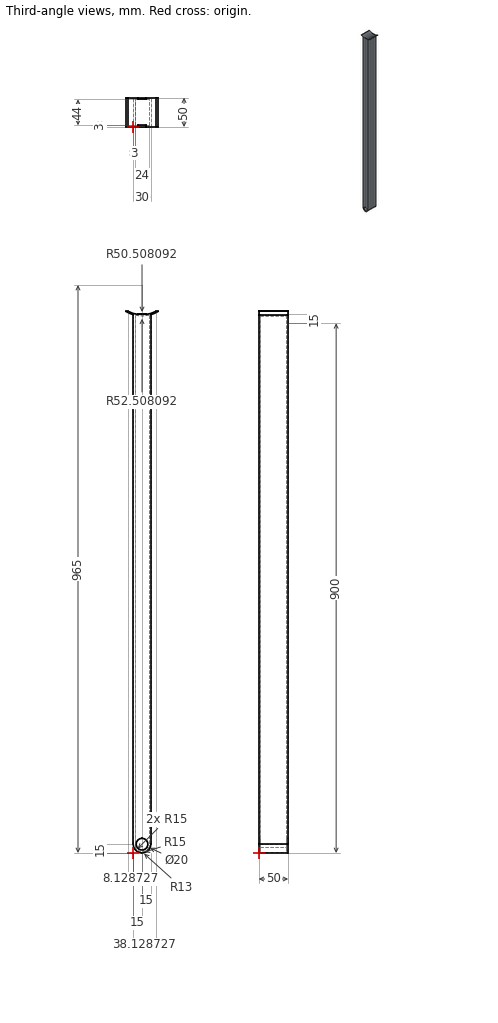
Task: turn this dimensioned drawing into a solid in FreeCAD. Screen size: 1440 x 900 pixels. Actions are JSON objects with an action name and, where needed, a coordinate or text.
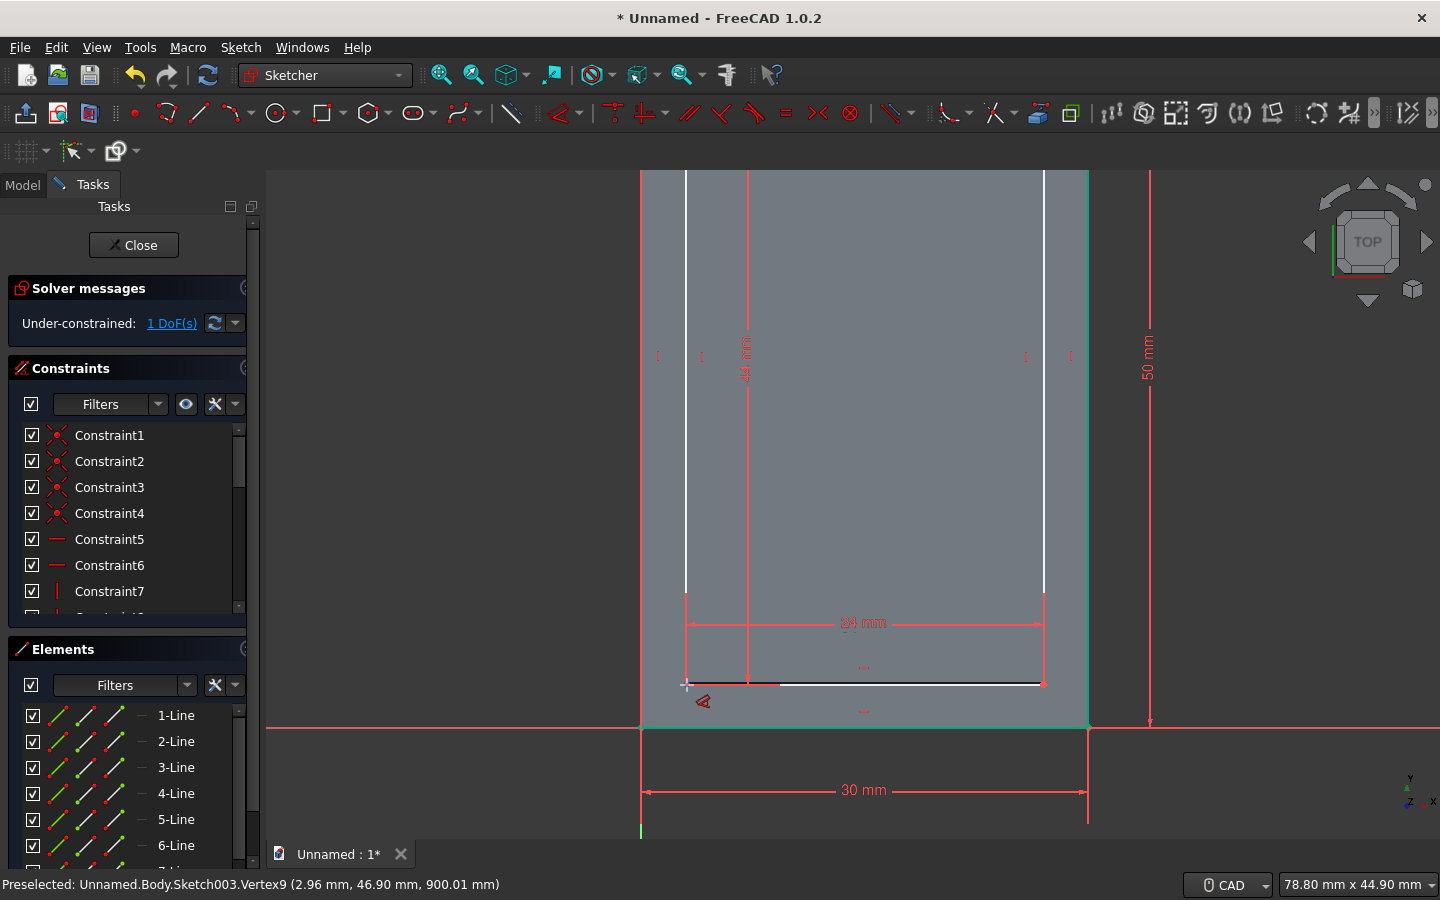
{"action": "left_click", "coordinate": [686, 685]}
{"action": "left_click", "coordinate": [607, 706]}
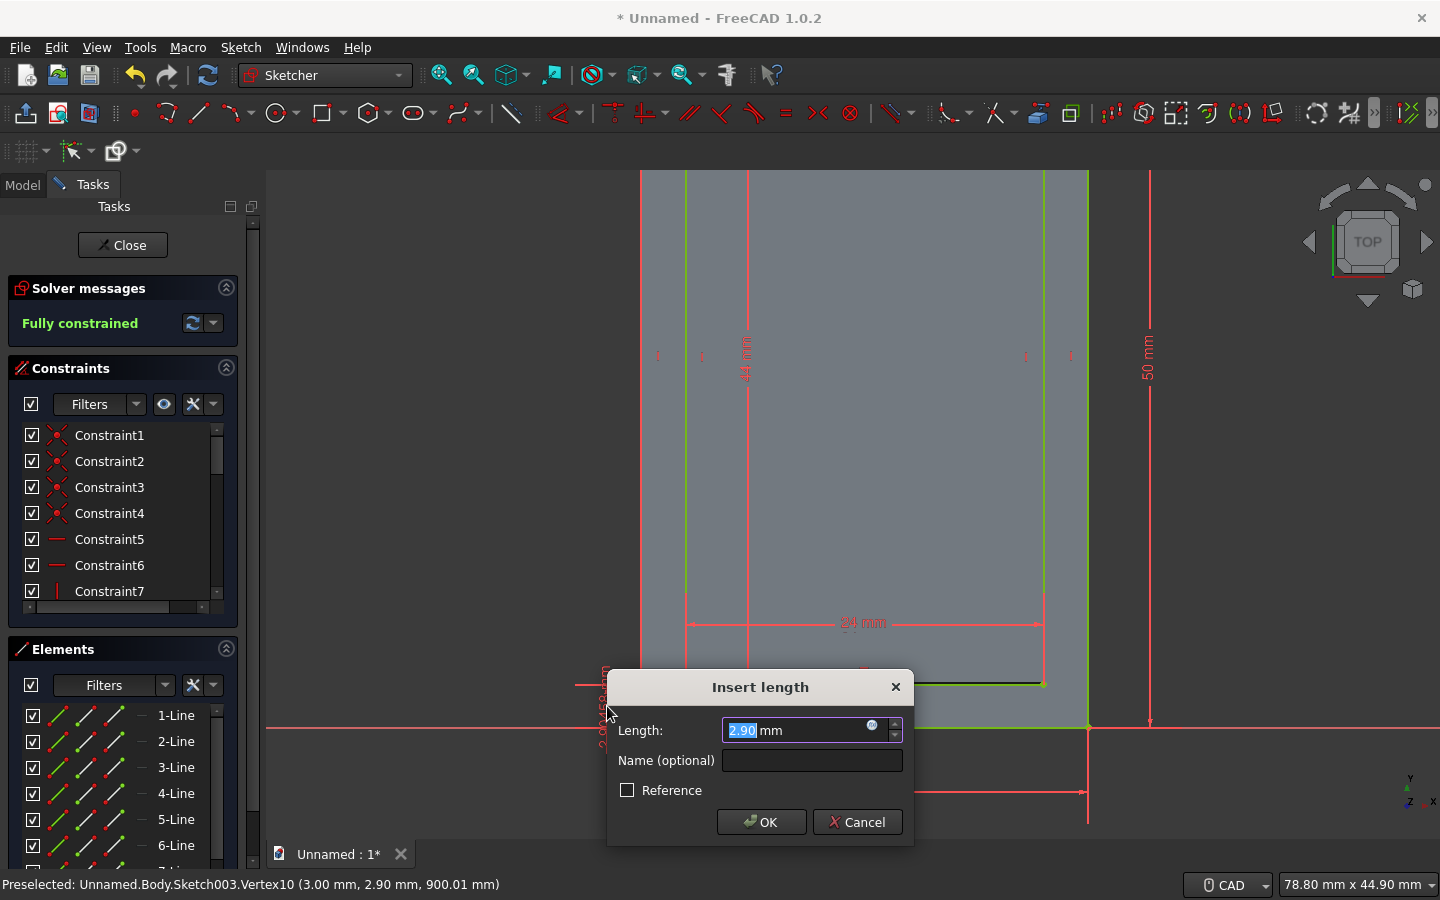
{"action": "type", "text": "3"}
{"action": "key", "text": "Return"}
{"action": "key", "text": "Escape"}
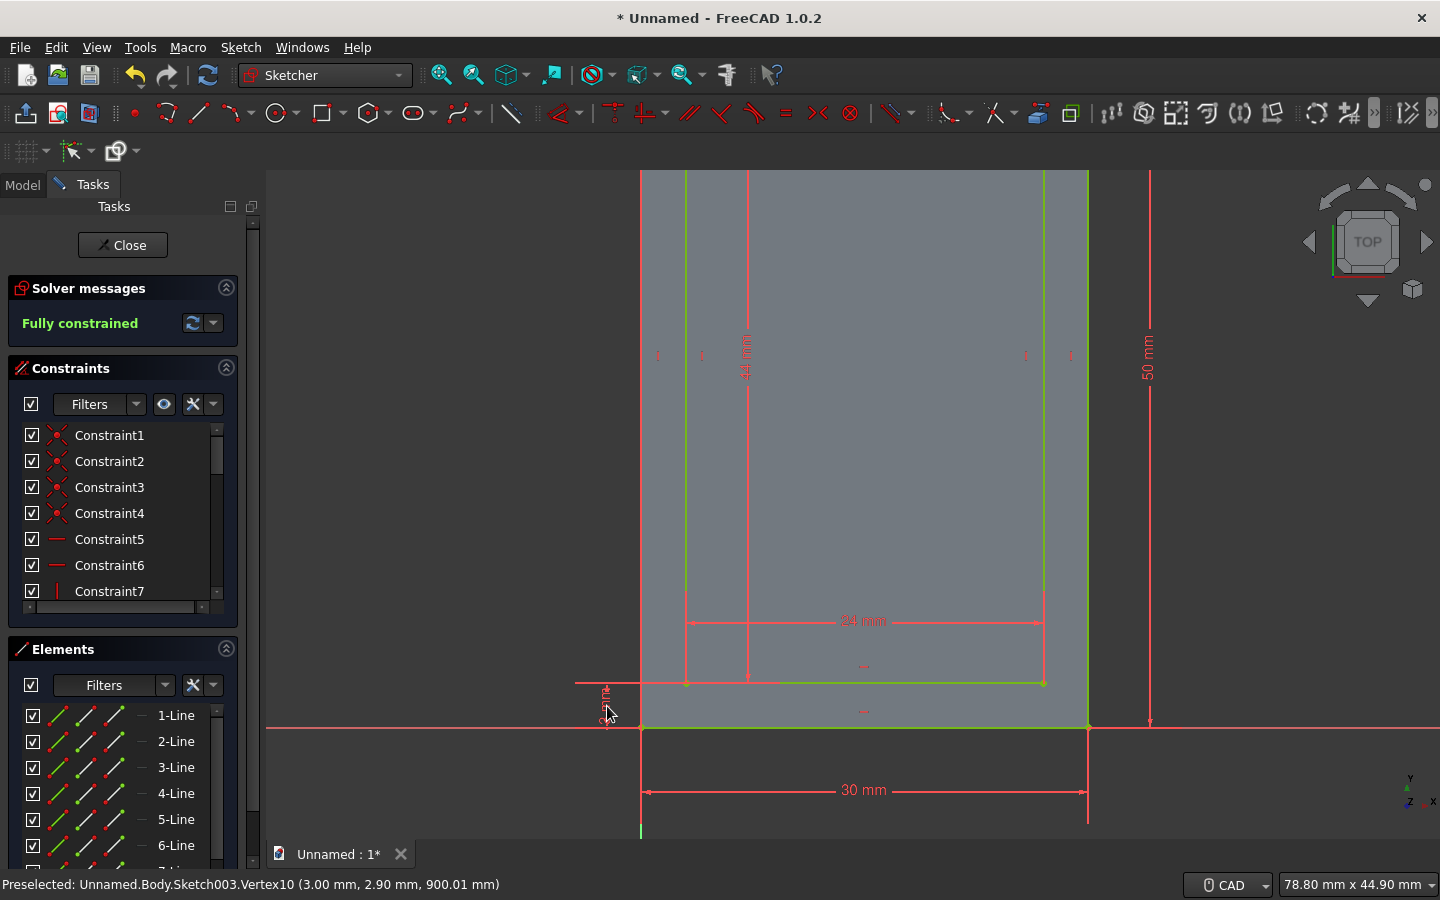
{"action": "left_click", "coordinate": [123, 245]}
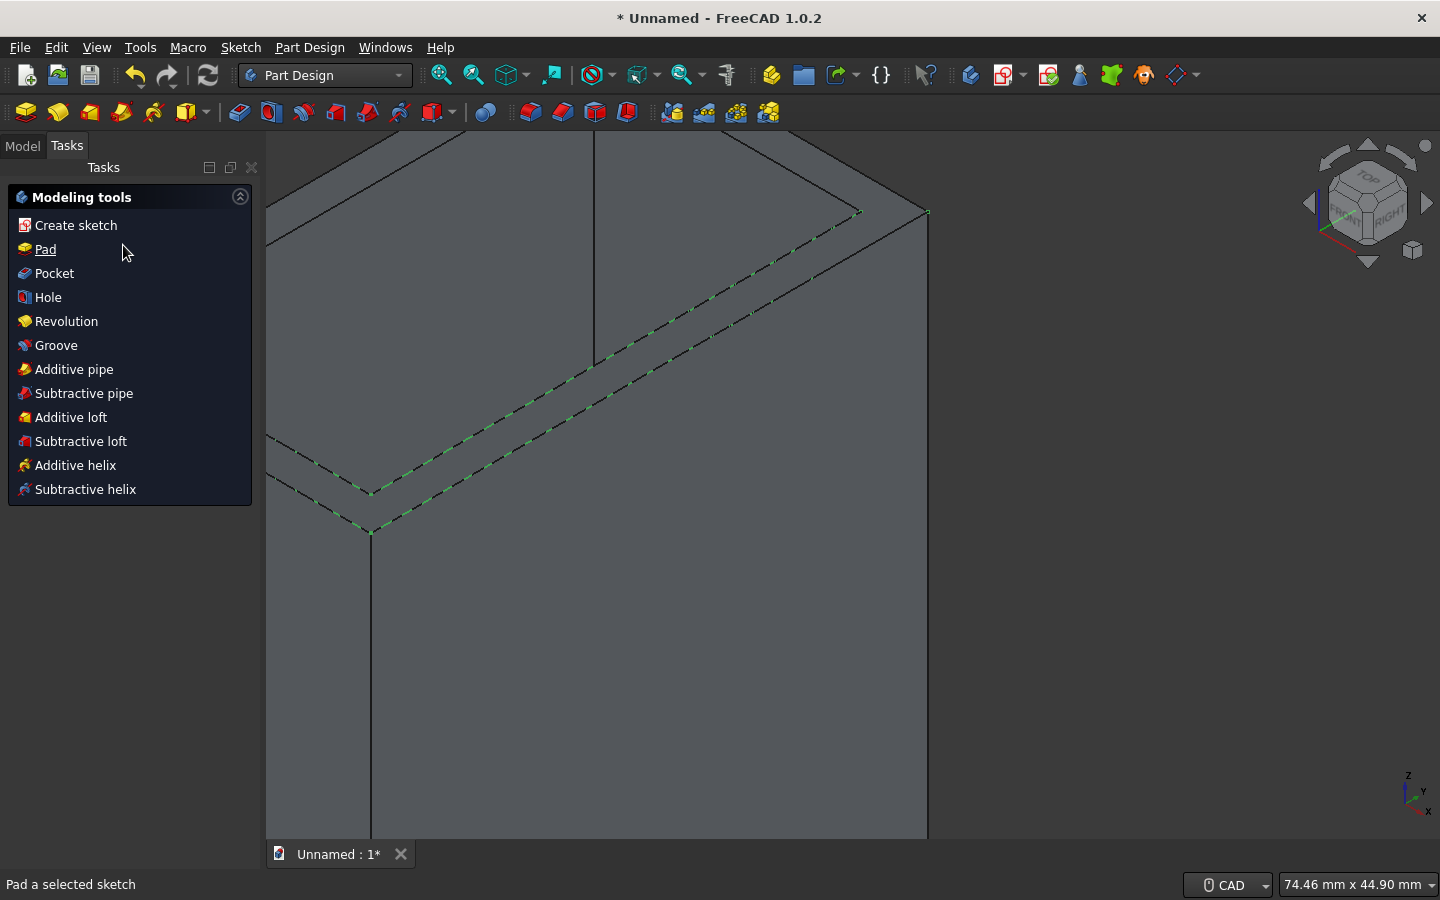
{"action": "left_click", "coordinate": [26, 112]}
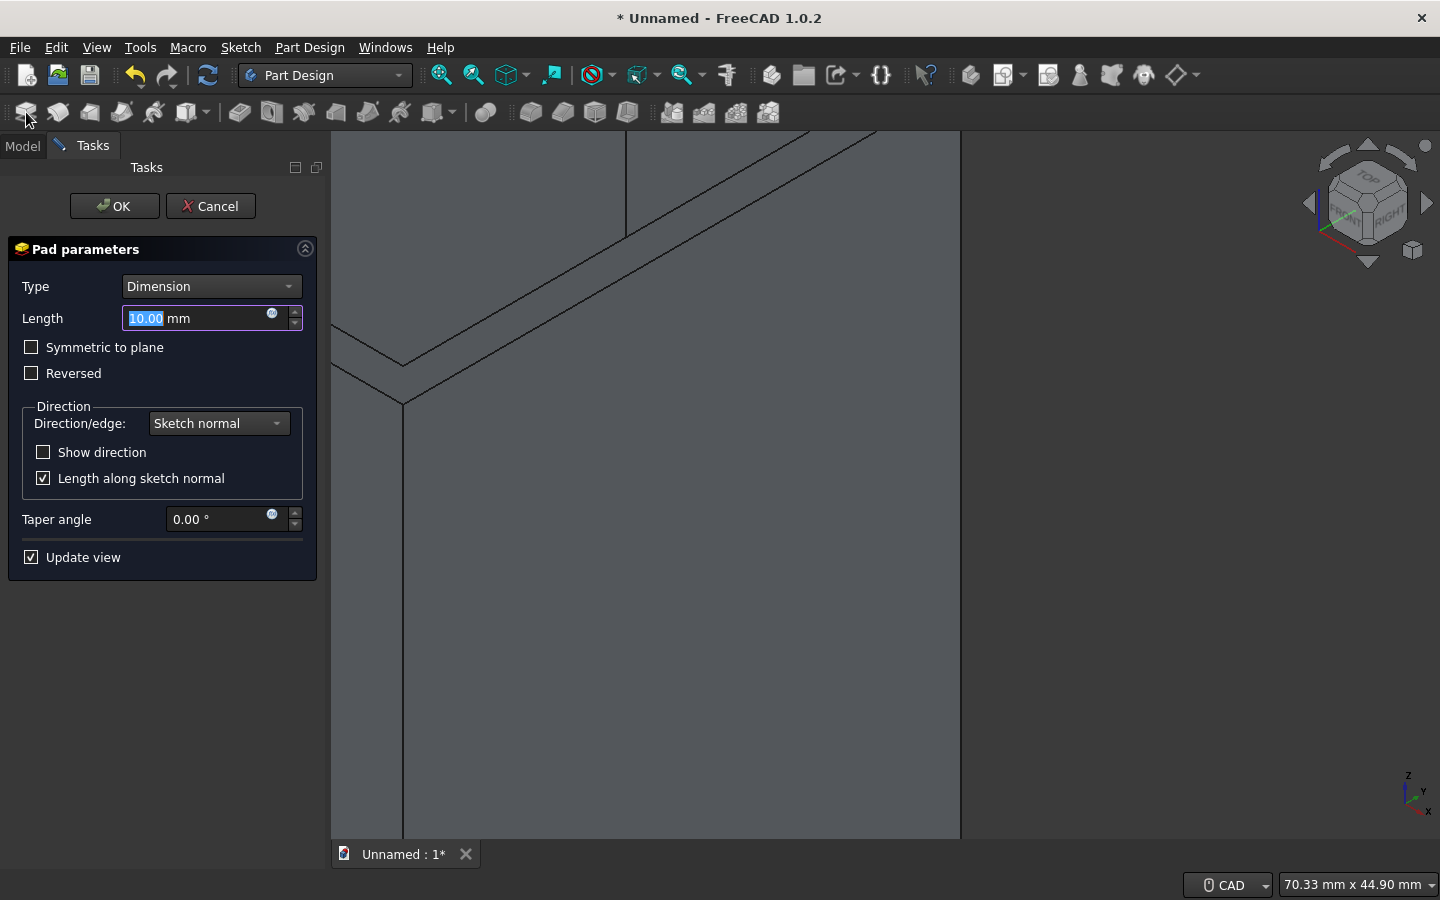
{"action": "type", "text": "15"}
{"action": "key", "text": "Tab"}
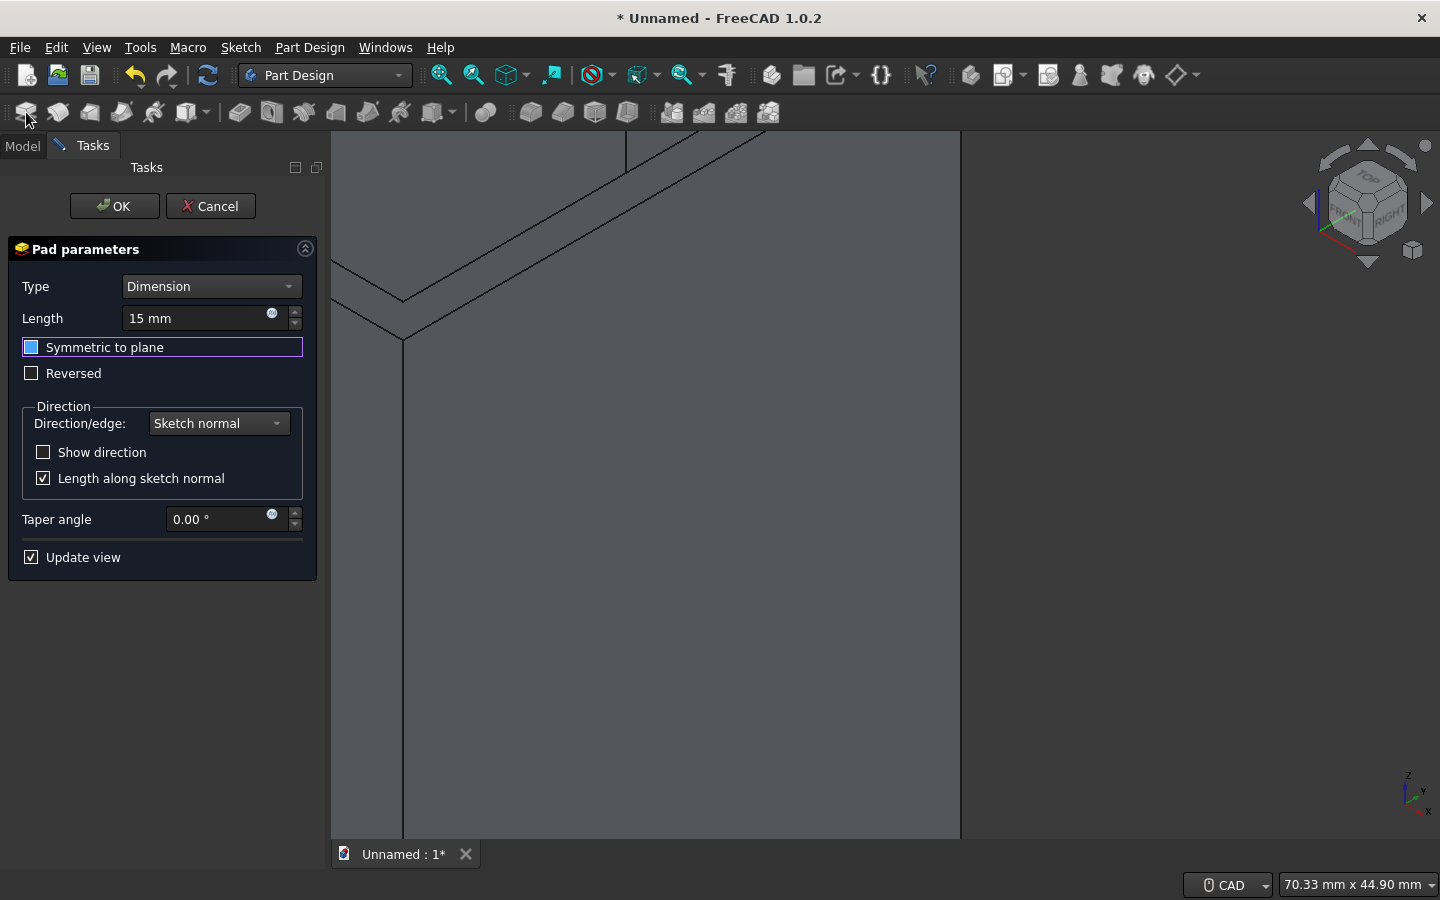
{"action": "left_click", "coordinate": [115, 206]}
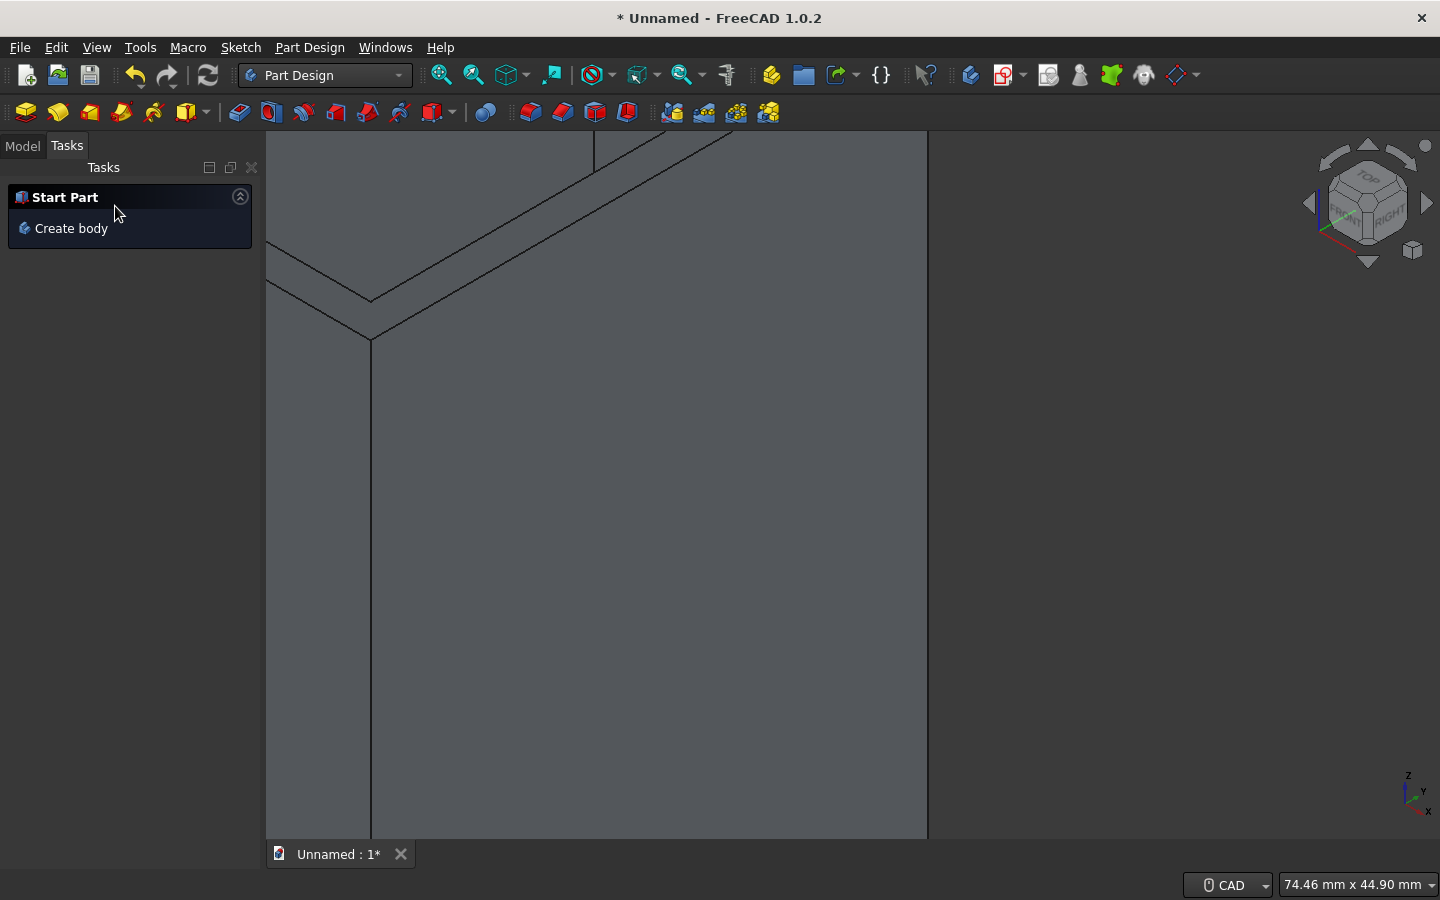
{"action": "left_click", "coordinate": [442, 76]}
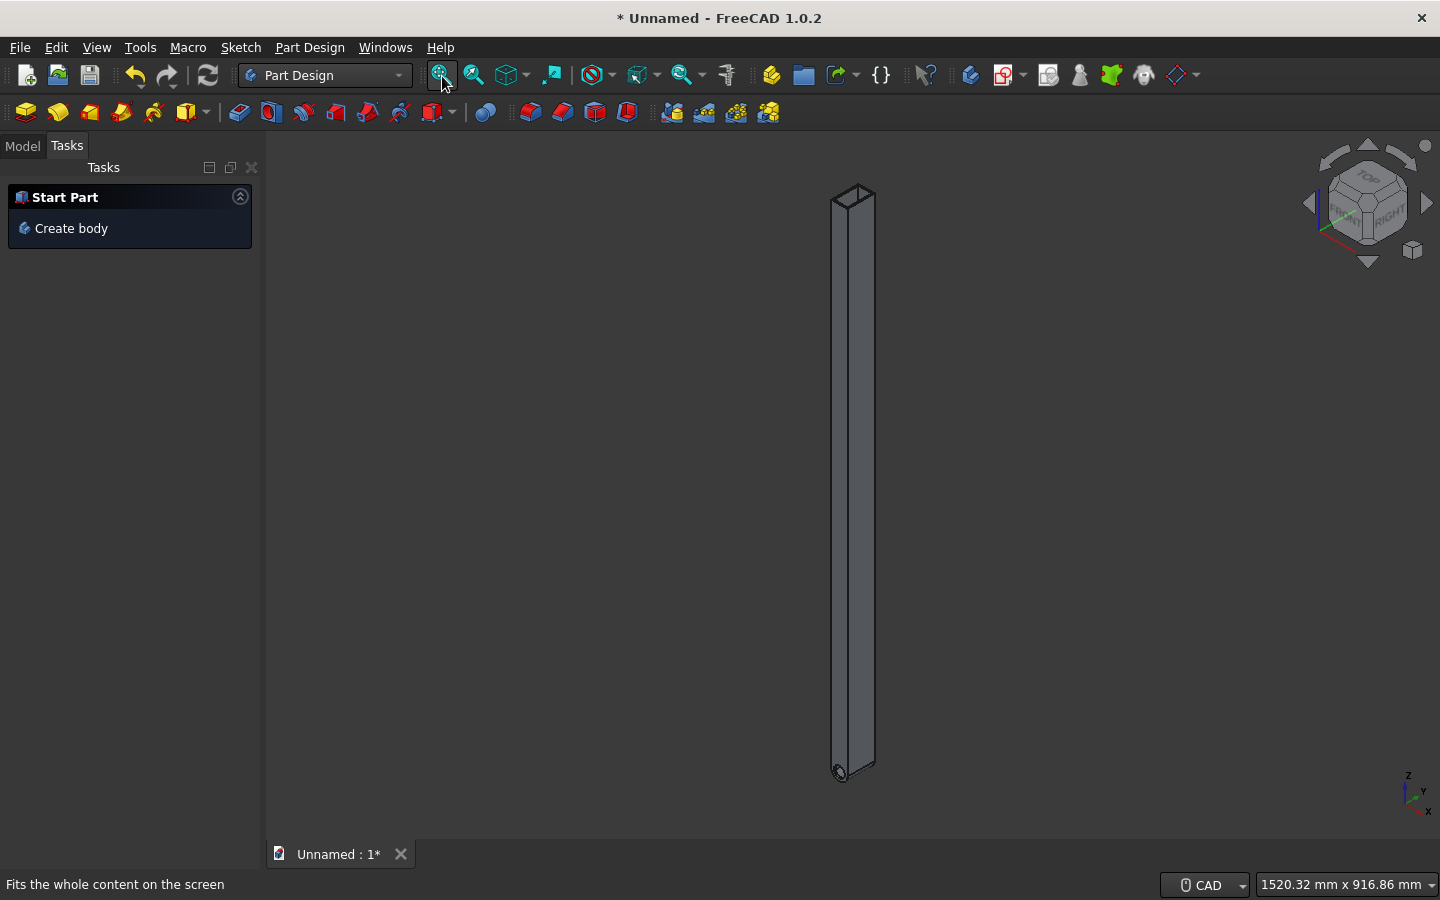
{"action": "key", "text": "4"}